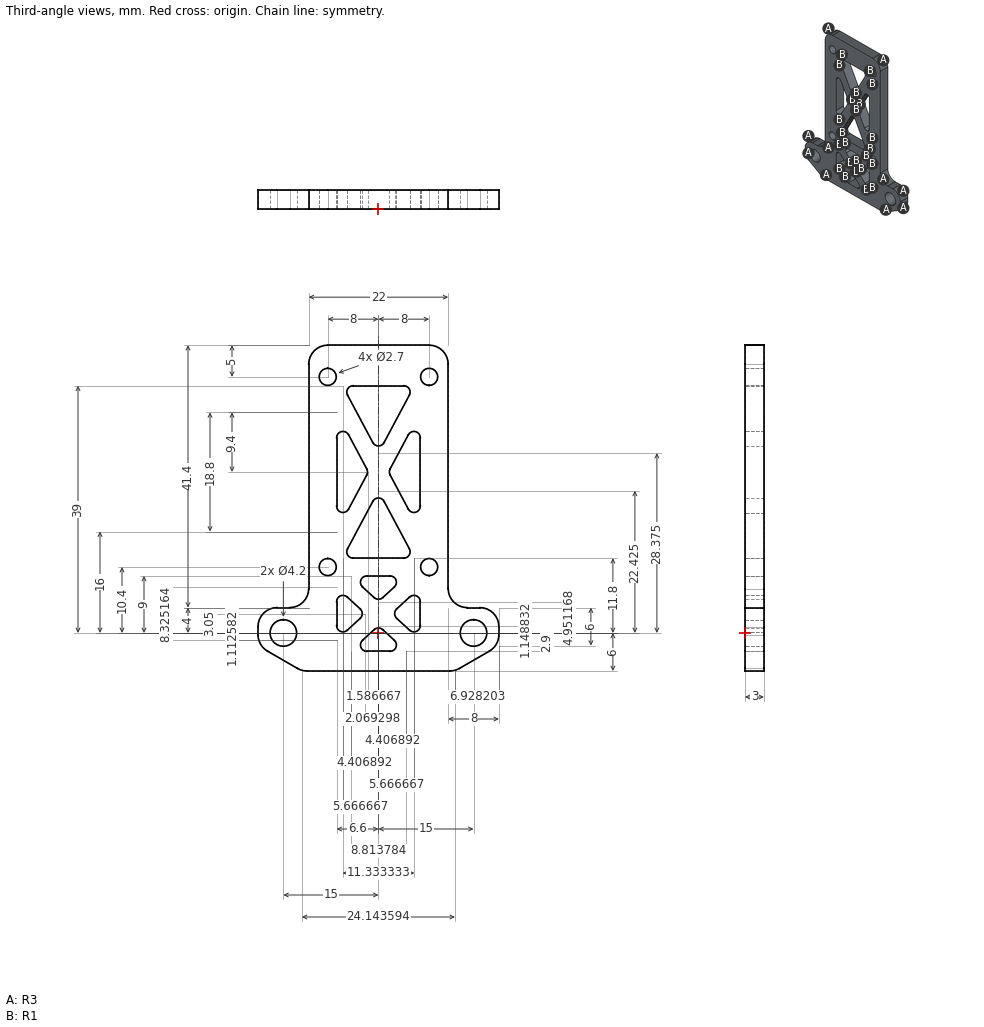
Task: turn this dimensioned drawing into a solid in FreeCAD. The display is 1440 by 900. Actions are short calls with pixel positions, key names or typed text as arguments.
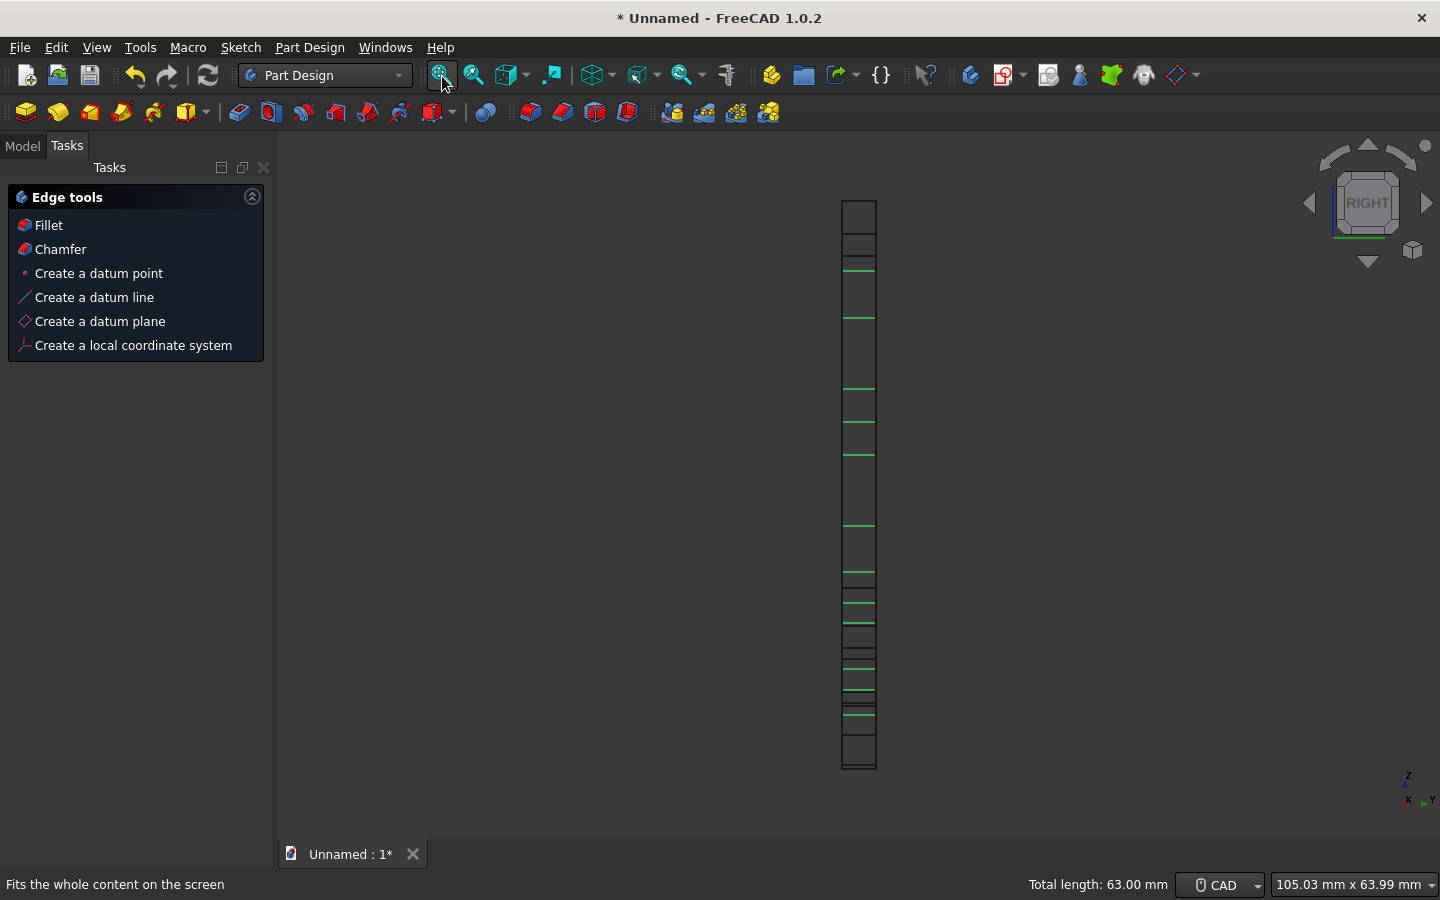
click(859, 647, ctrl)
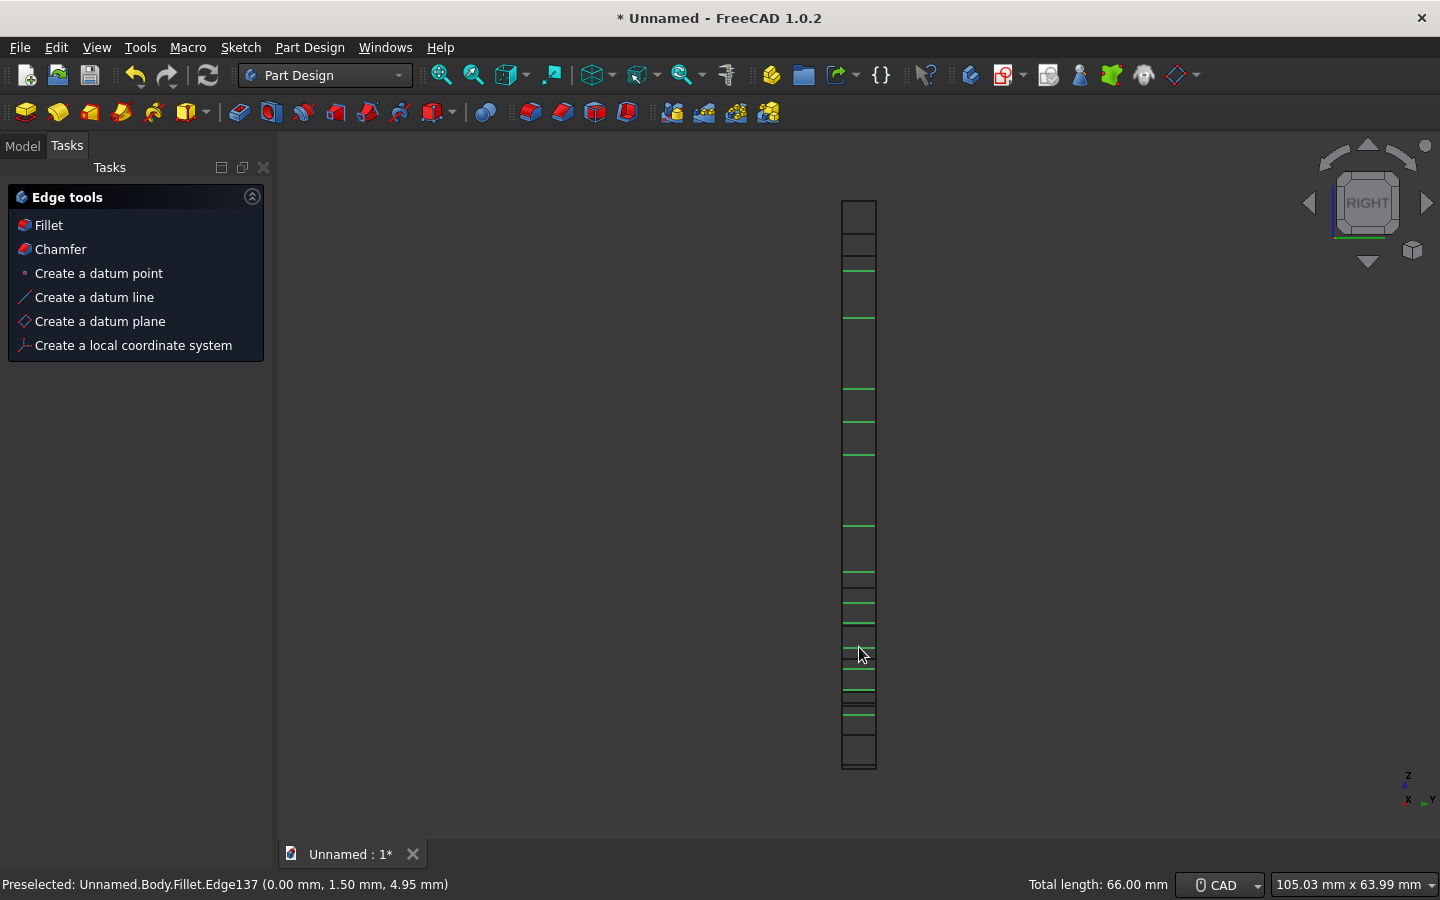
scroll(859, 714, up, 6)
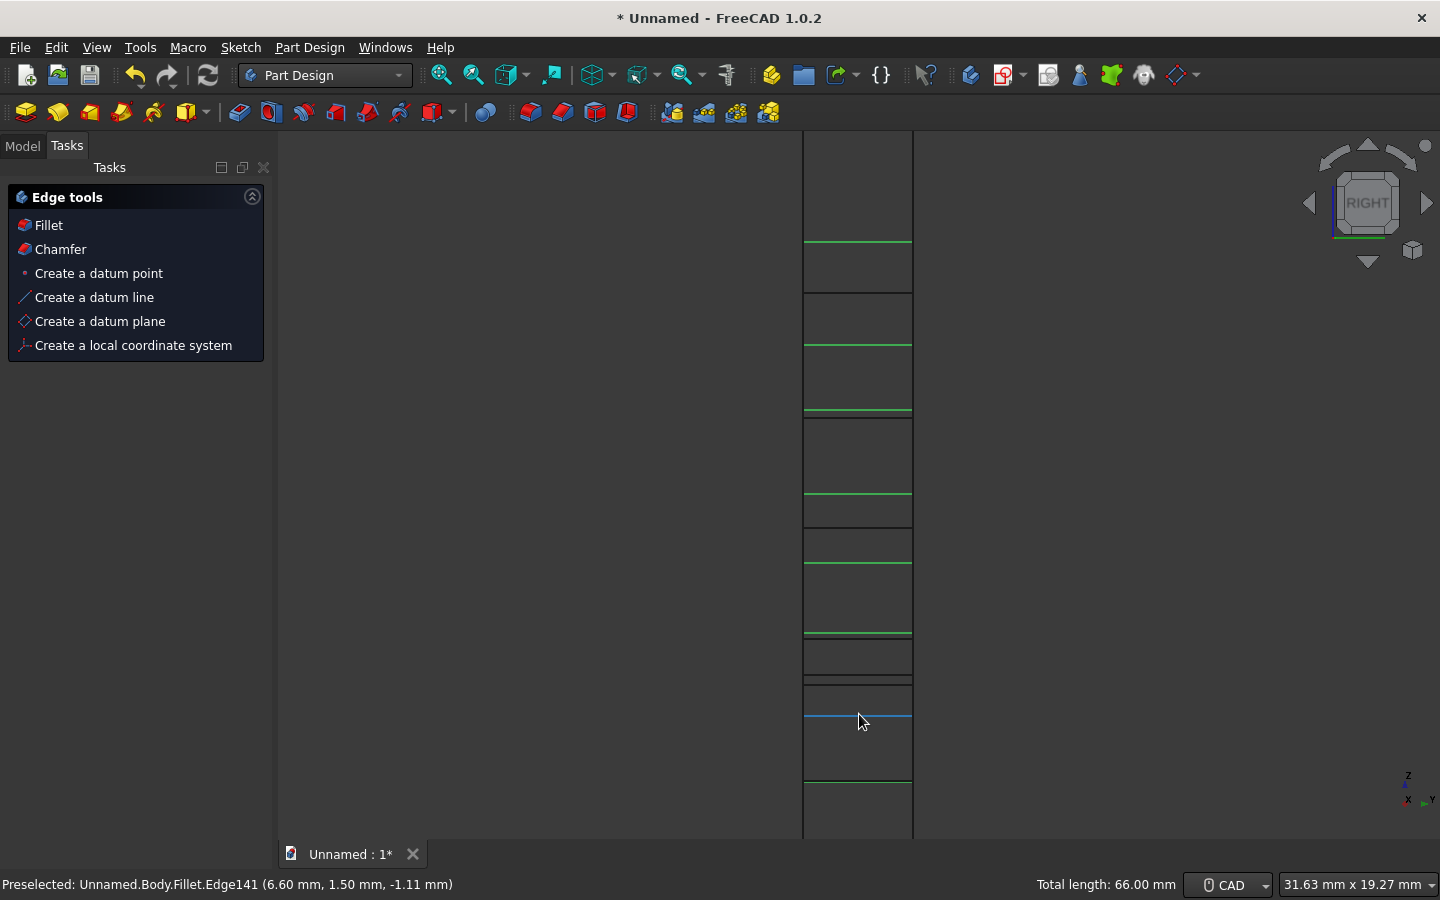
click(442, 76)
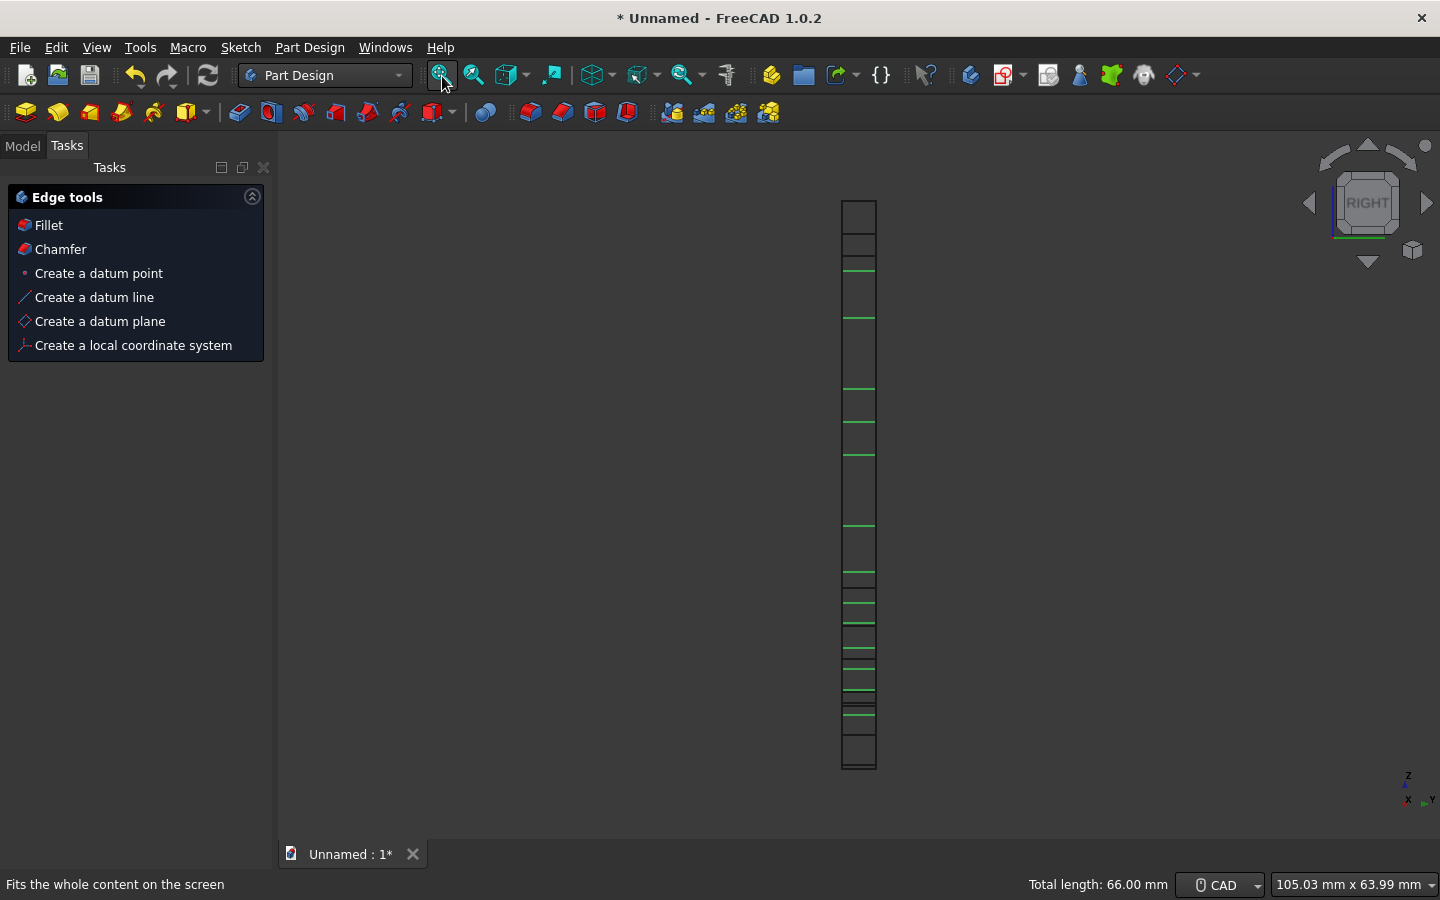
key(5)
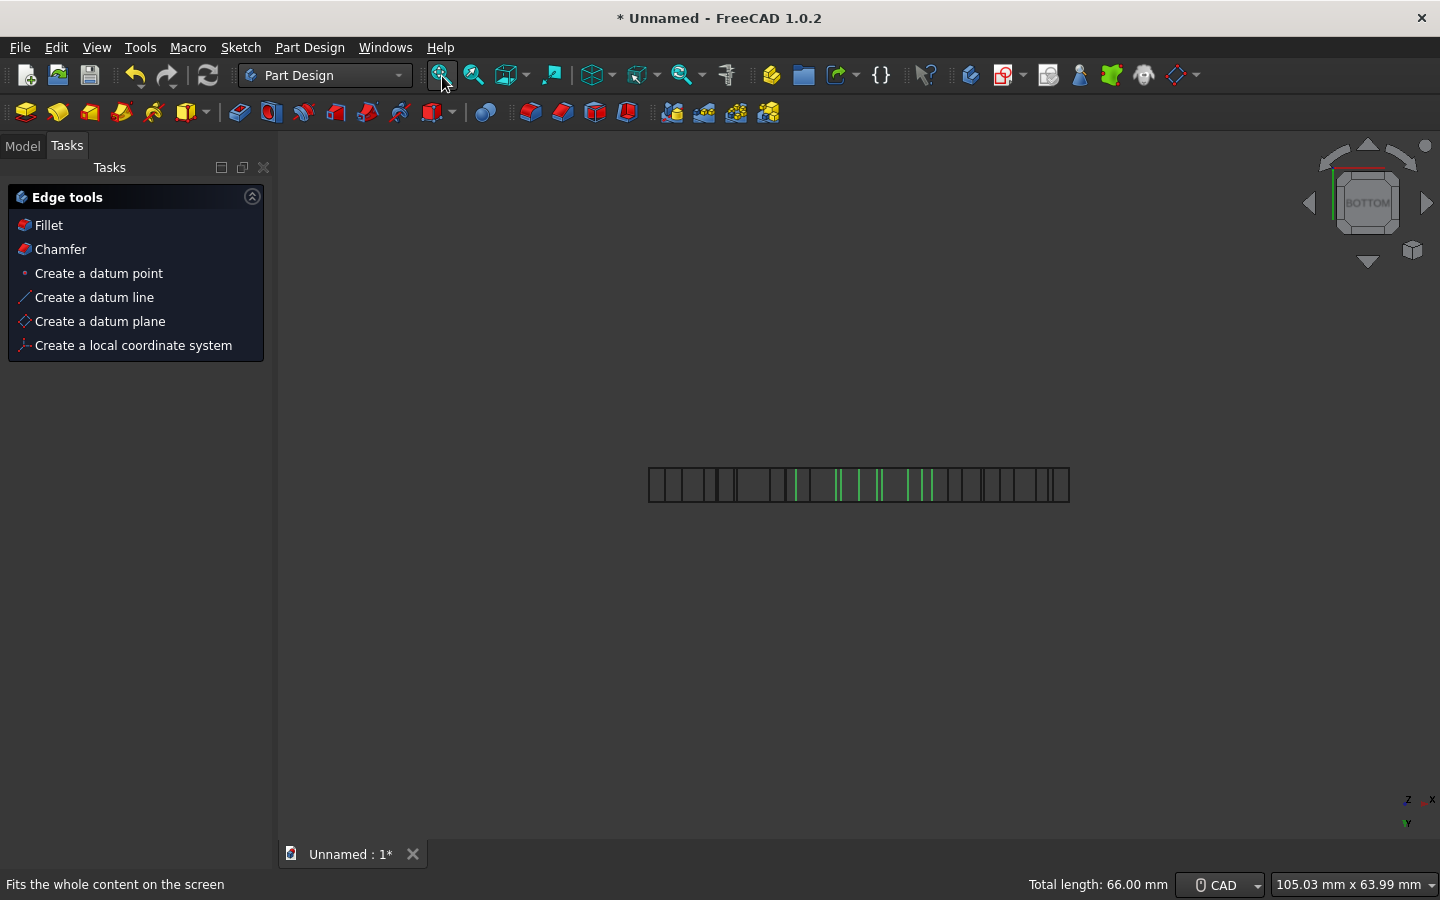
click(442, 76)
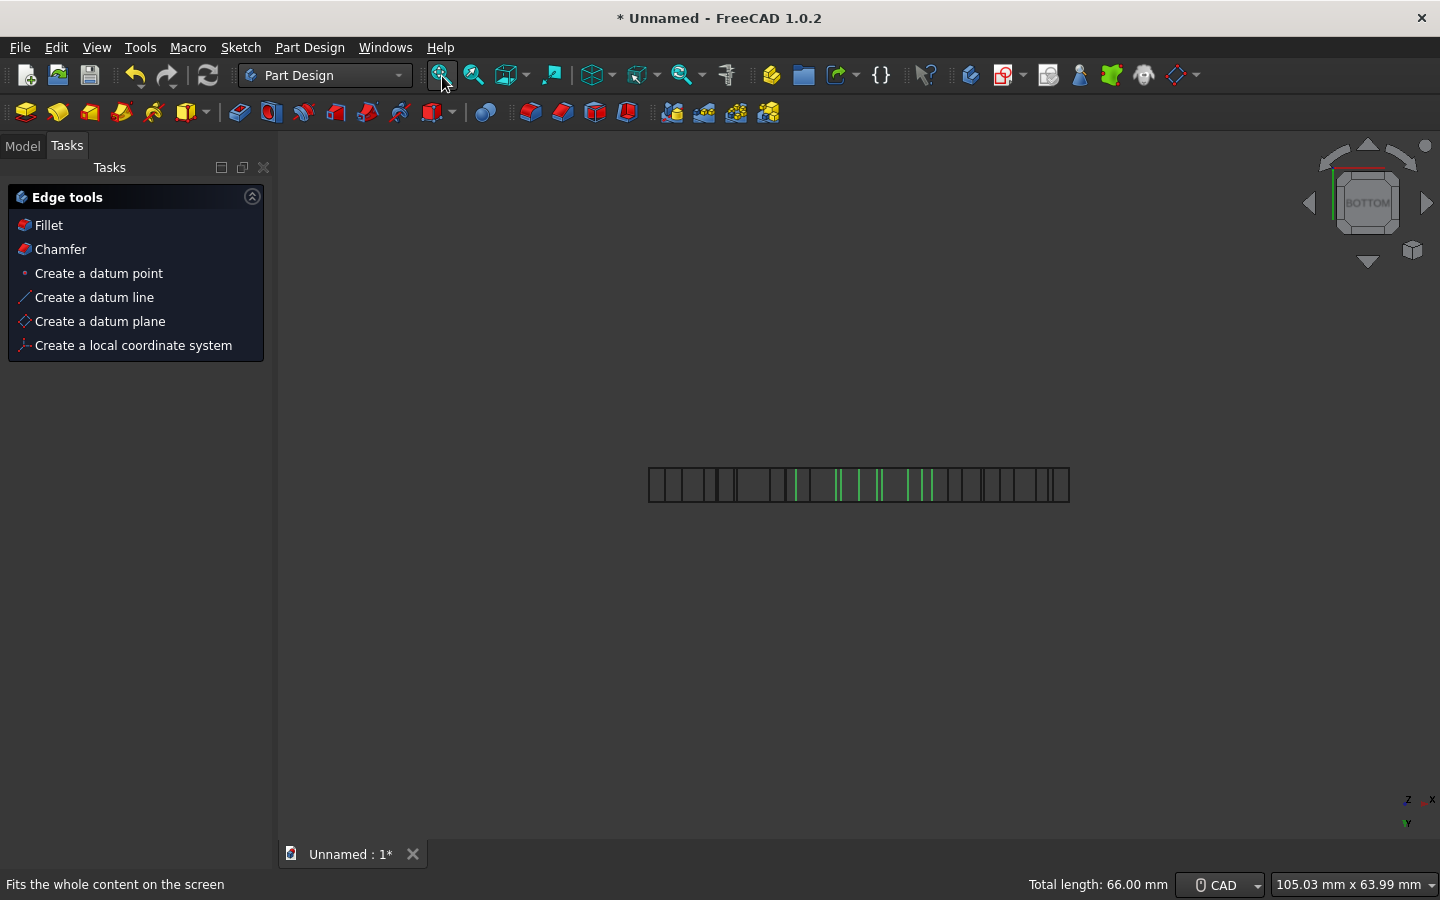
click(786, 484, ctrl)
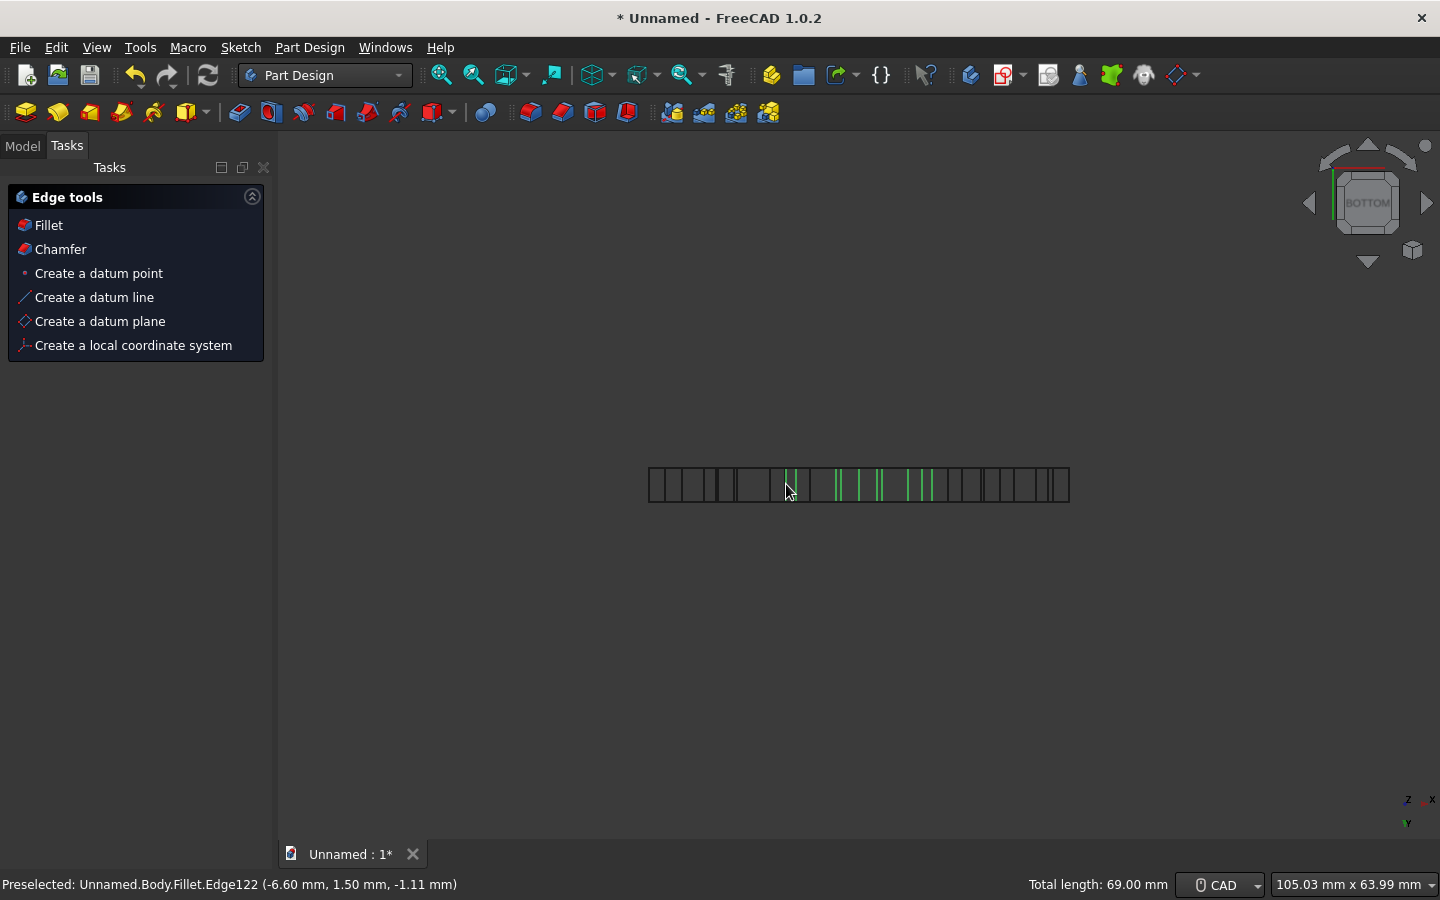
click(810, 484, ctrl)